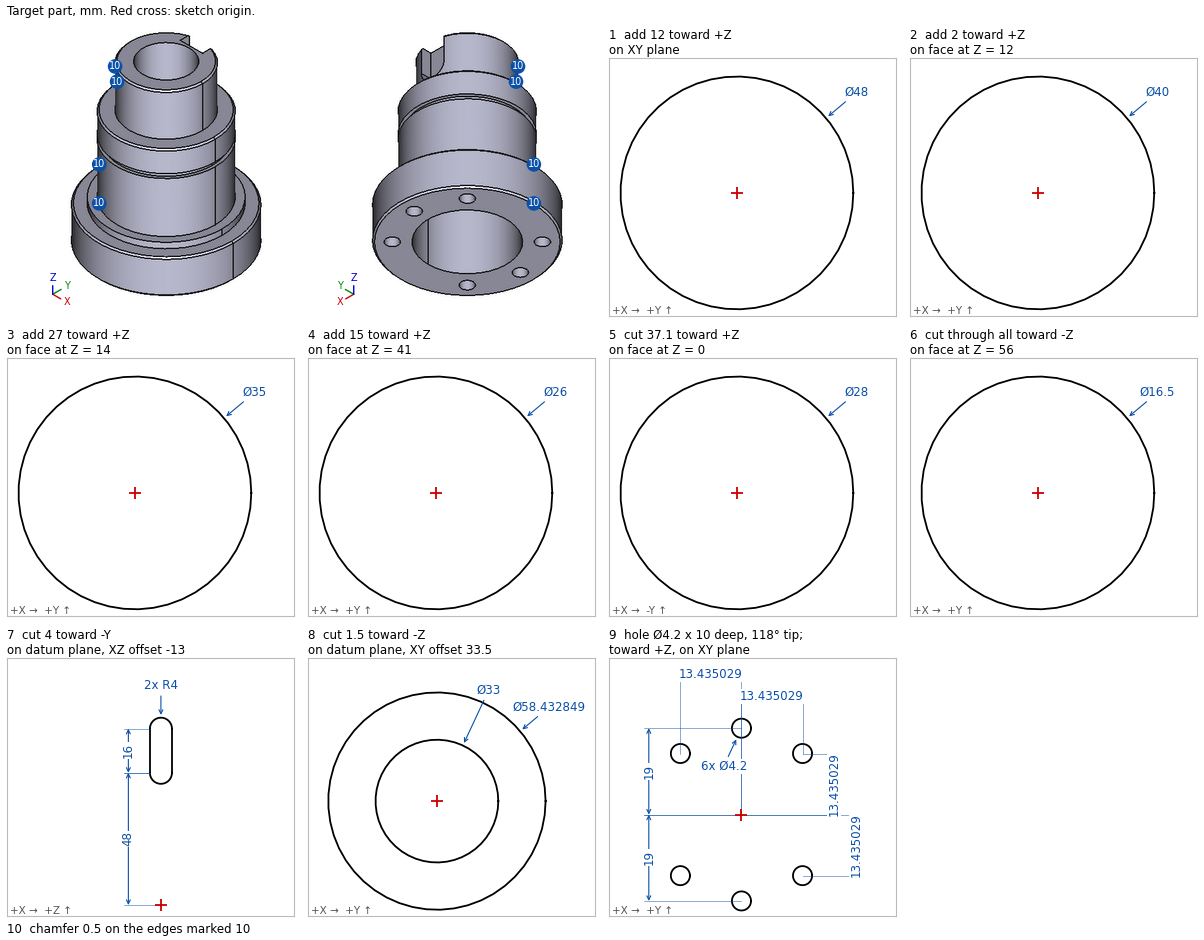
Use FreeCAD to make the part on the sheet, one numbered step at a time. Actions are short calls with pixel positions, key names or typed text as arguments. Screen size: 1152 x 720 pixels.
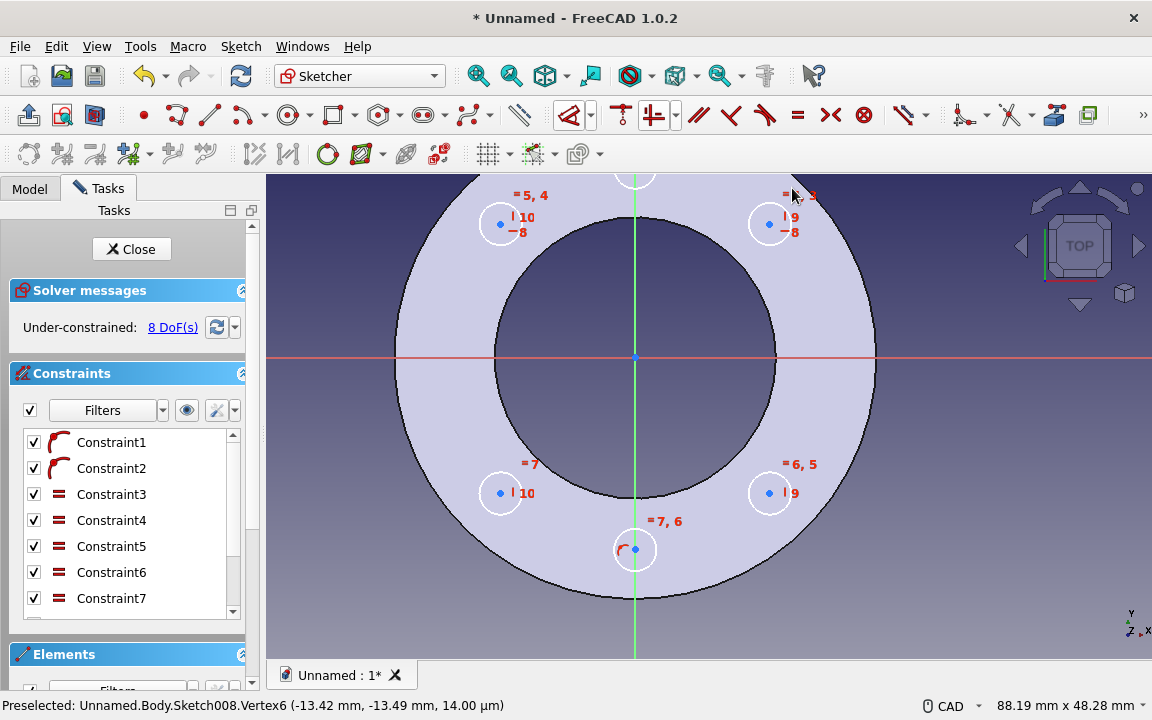
click(770, 494)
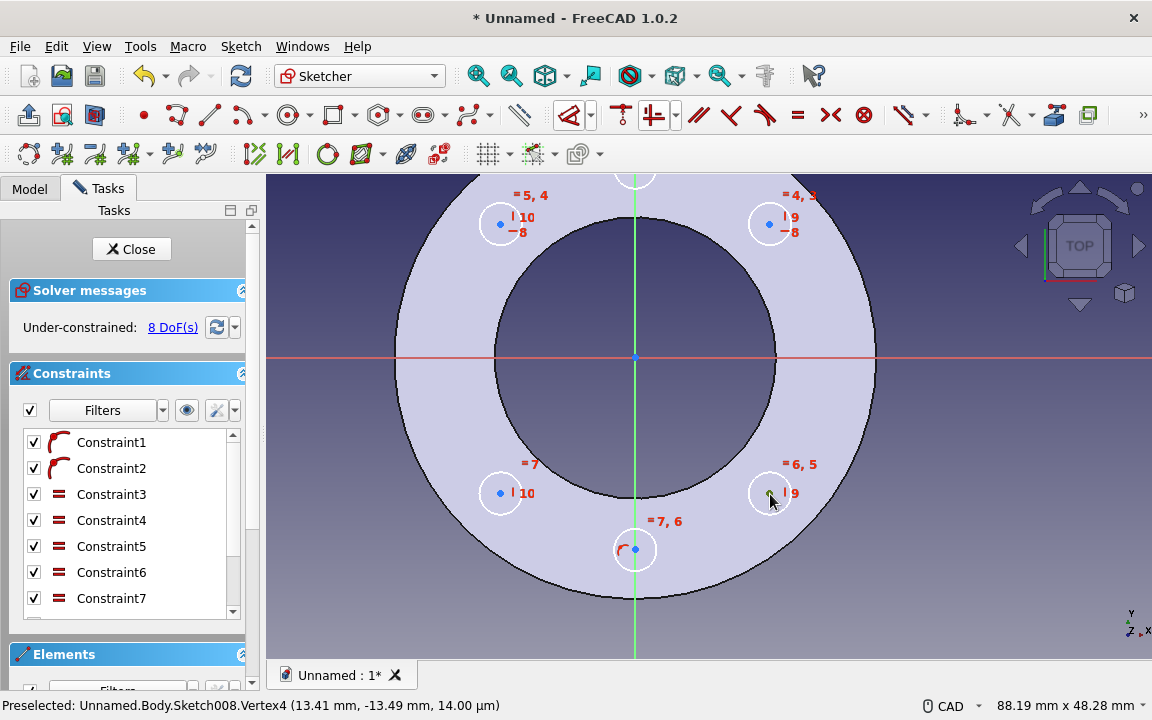
click(501, 494)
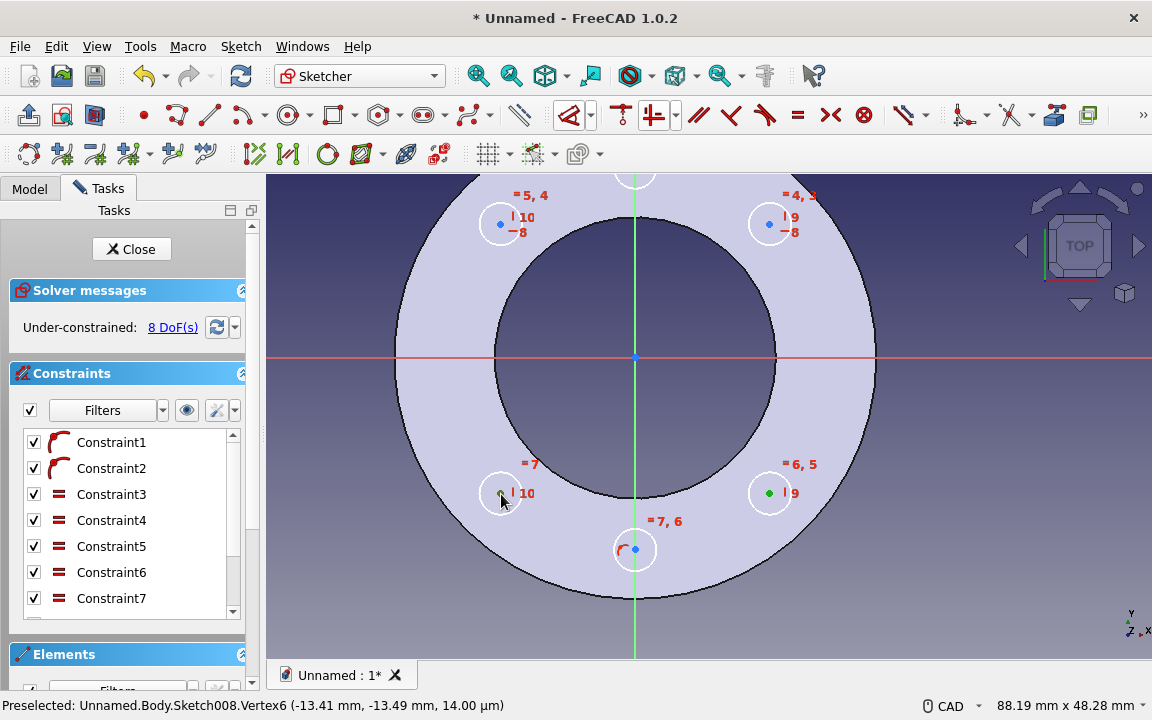
key(h)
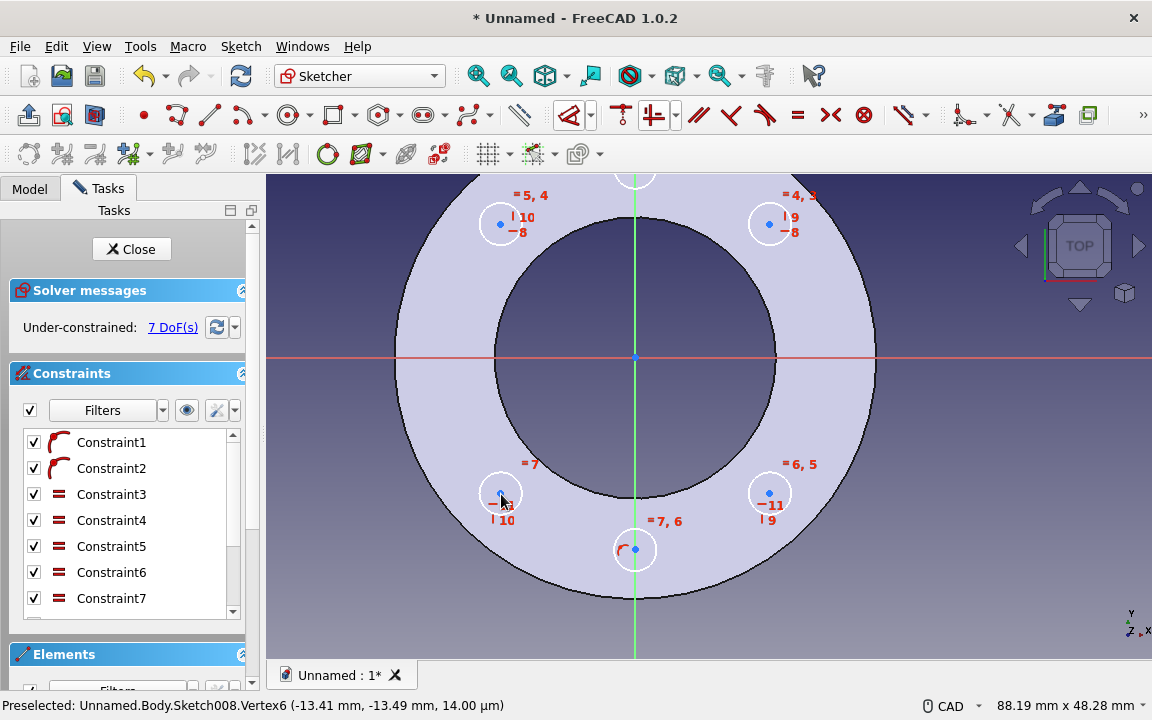
scroll(651, 535, down, 2)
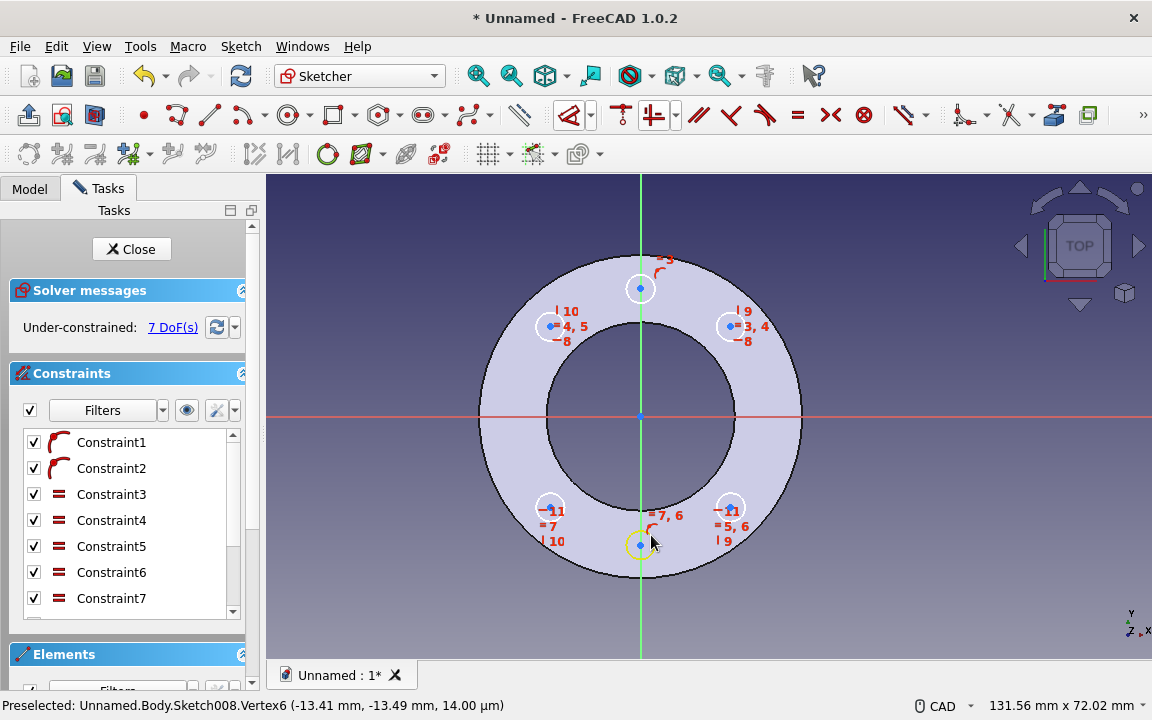
scroll(651, 279, up, 2)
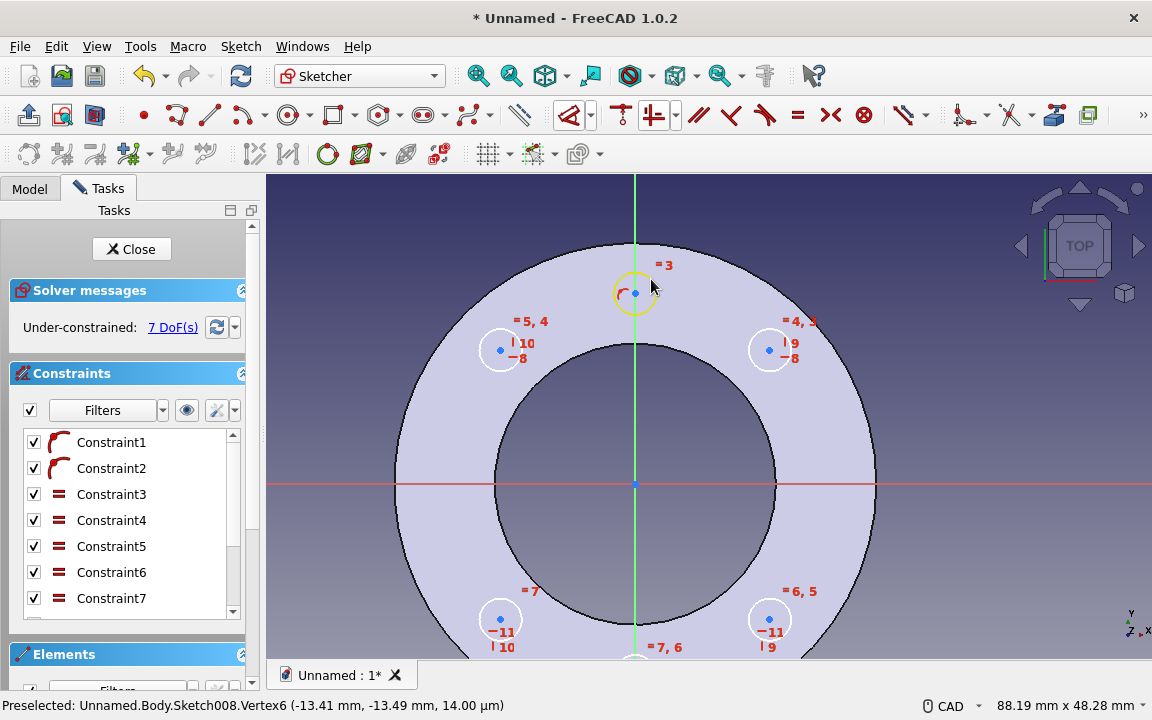
click(650, 279)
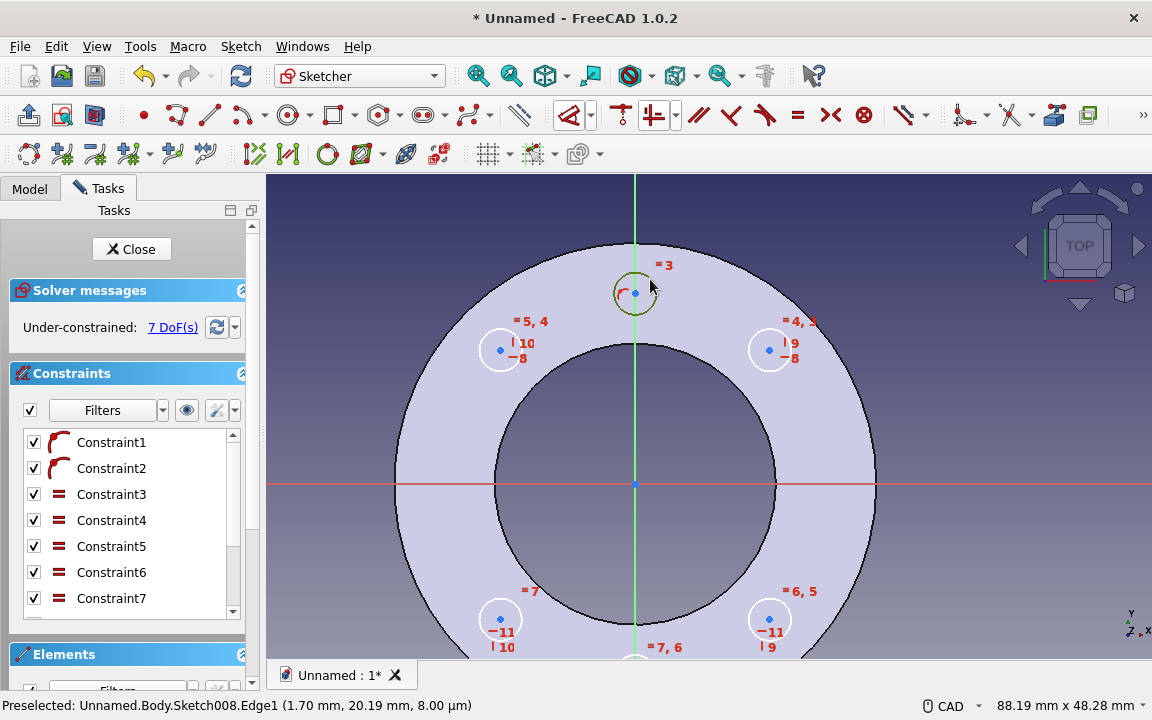
key(k)
key(o)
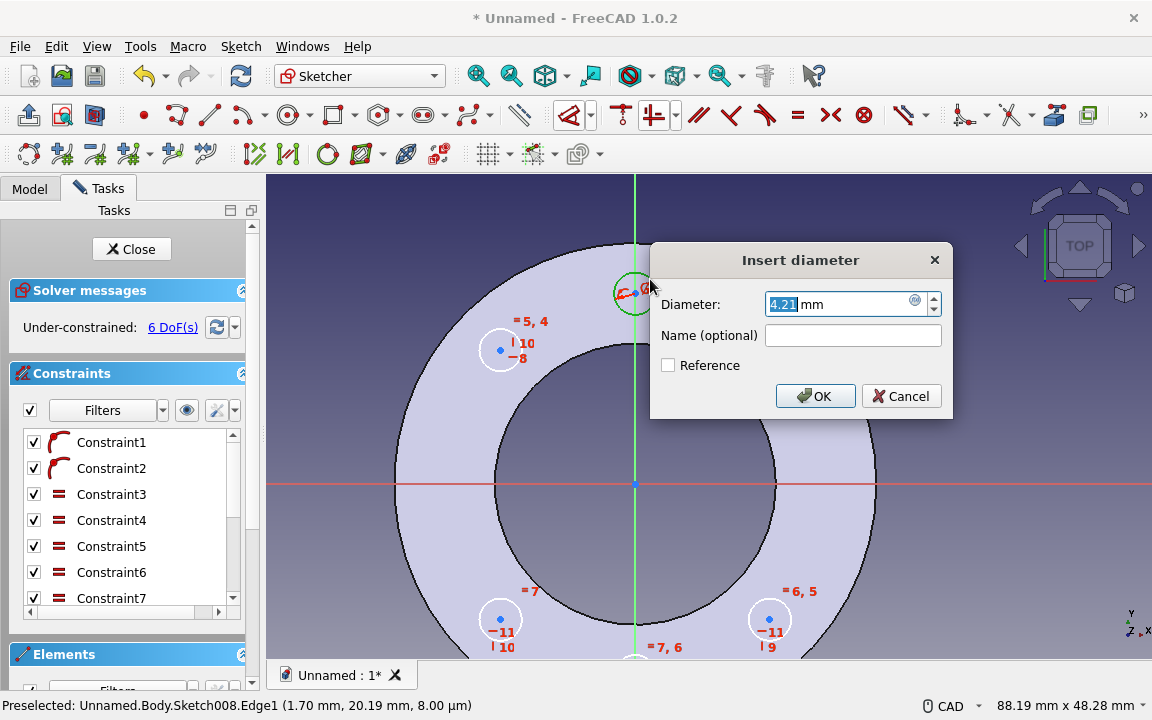
text(4.2)
key(Return)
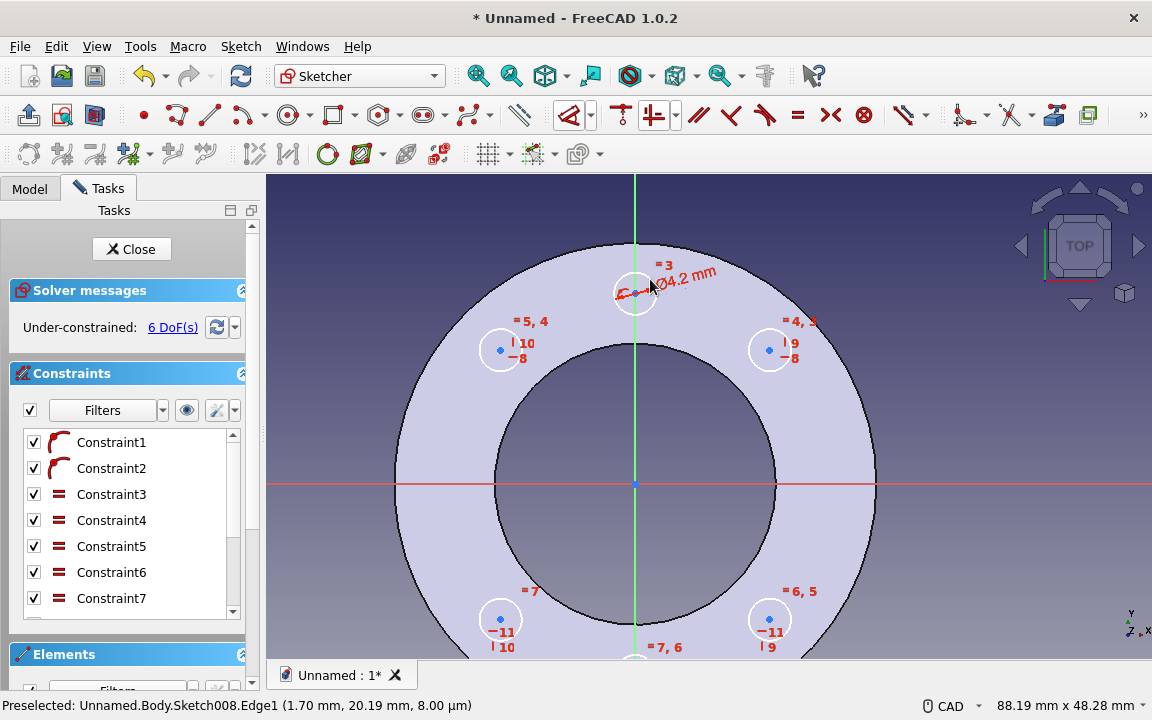
click(635, 294)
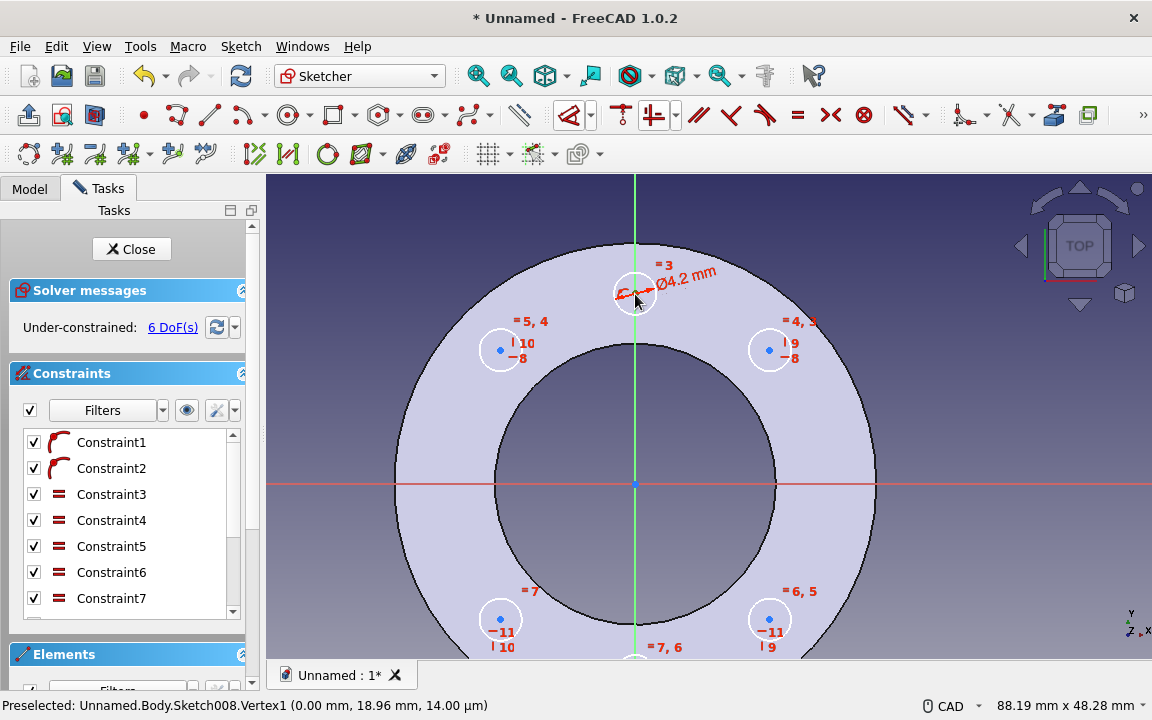
key(i)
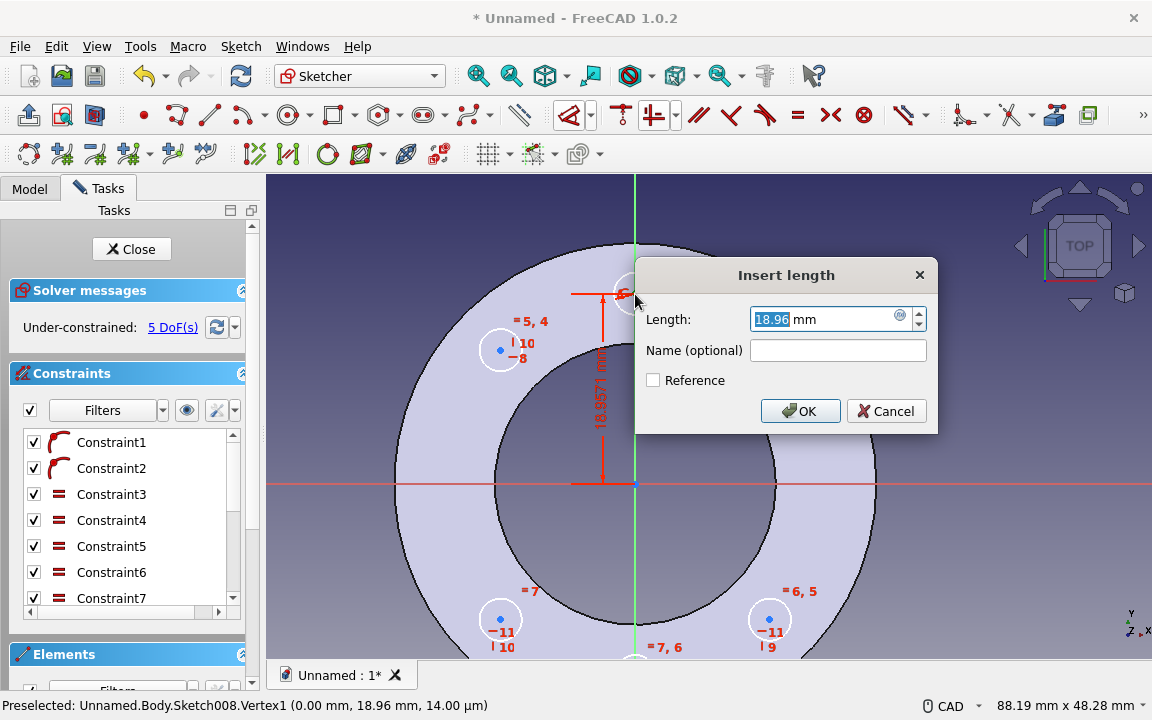
text(19)
key(Return)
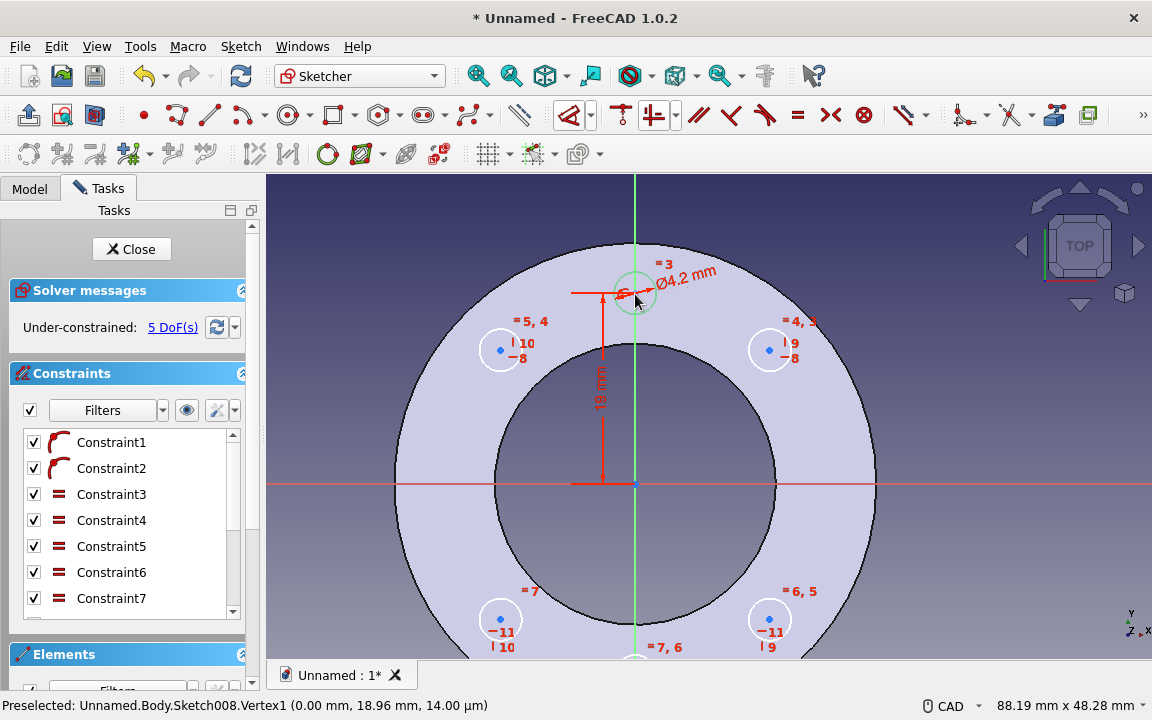
scroll(651, 279, down, 2)